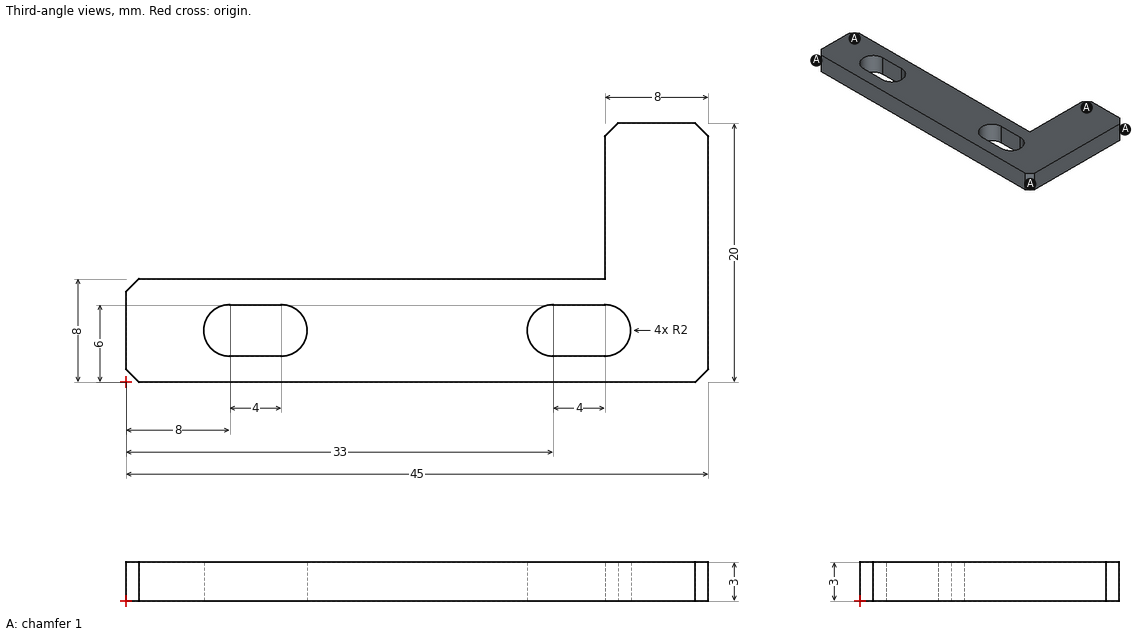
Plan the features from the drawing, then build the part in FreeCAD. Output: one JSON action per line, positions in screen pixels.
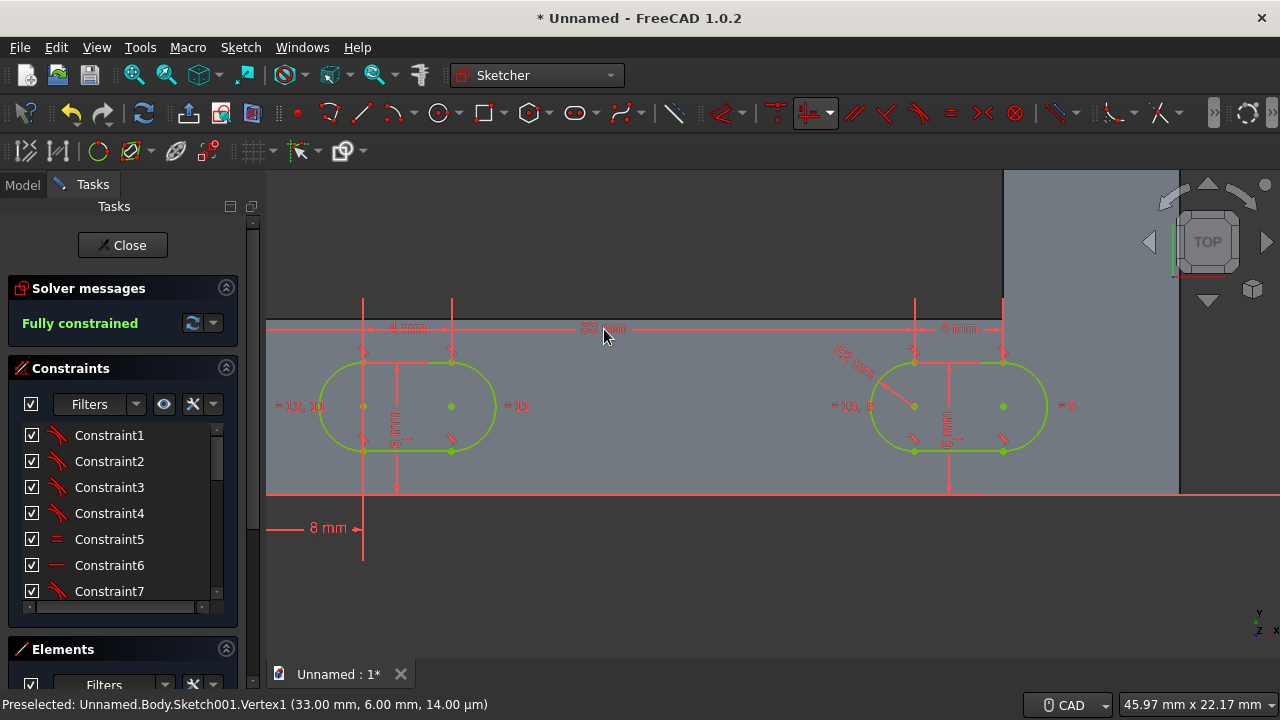
{"action": "left_click", "coordinate": [123, 245]}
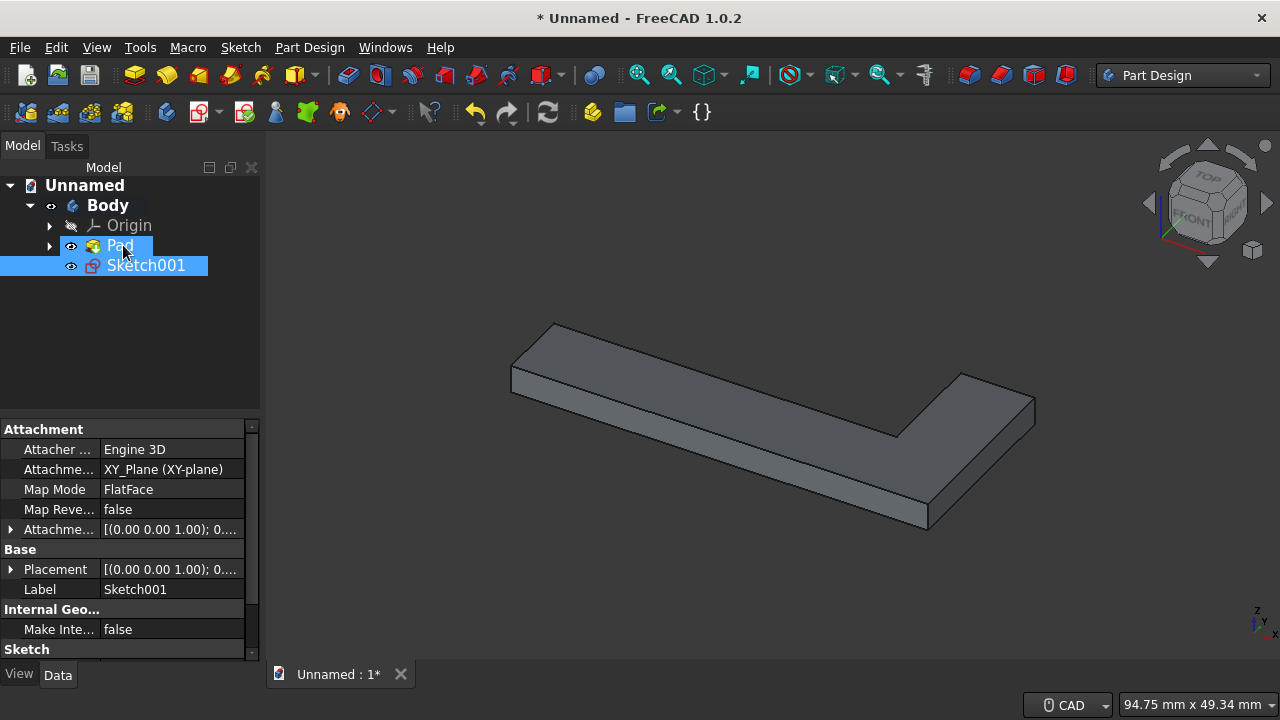
{"action": "left_click", "coordinate": [350, 76]}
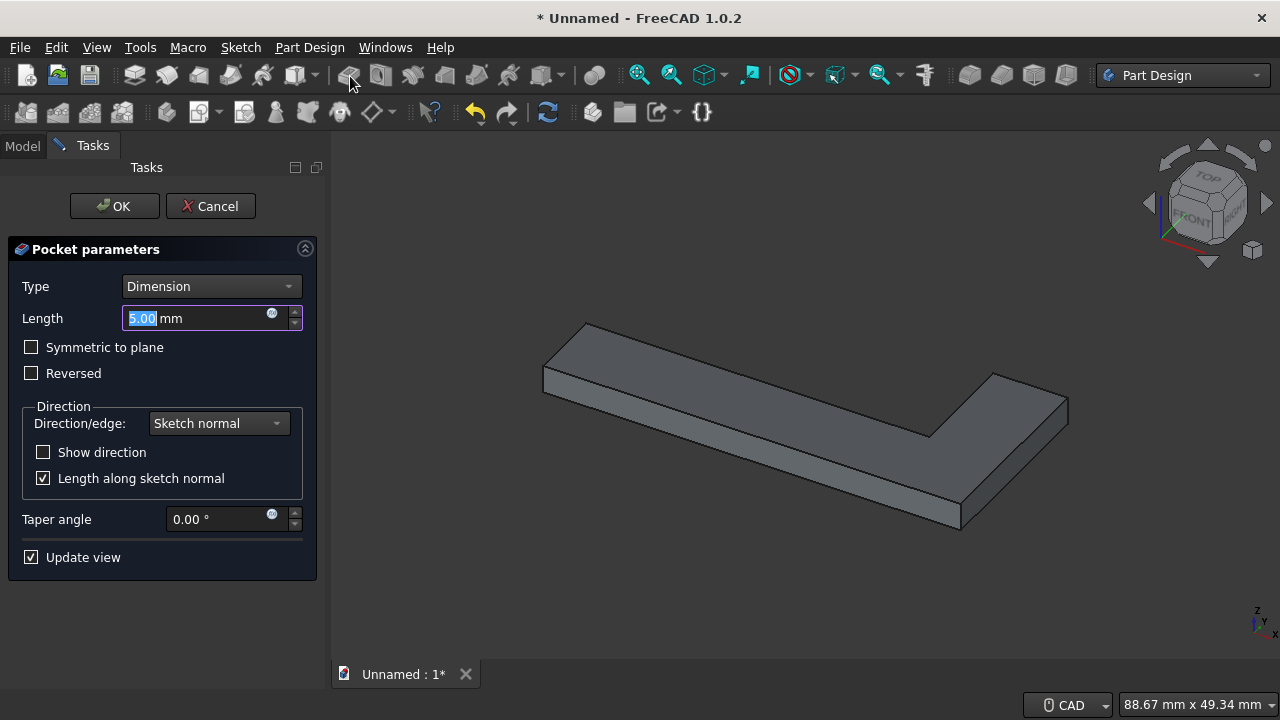
{"action": "type", "text": "3"}
{"action": "key", "text": "Tab"}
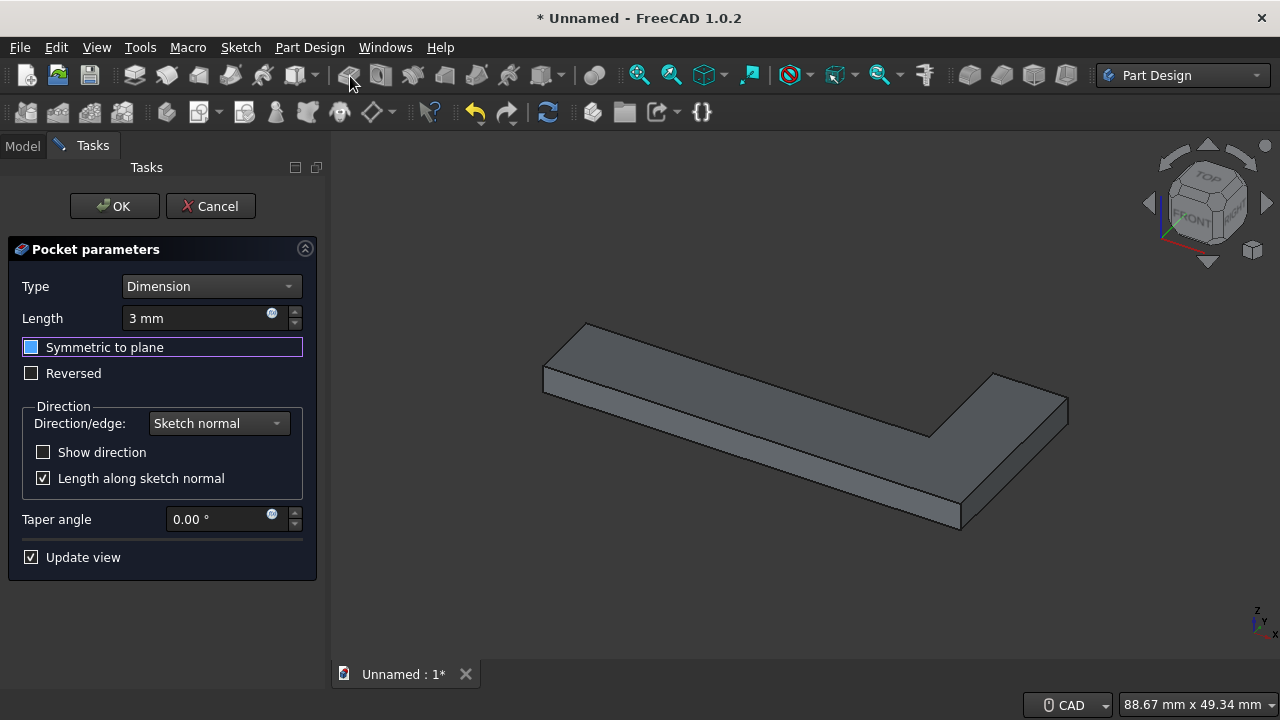
{"action": "left_click", "coordinate": [30, 373]}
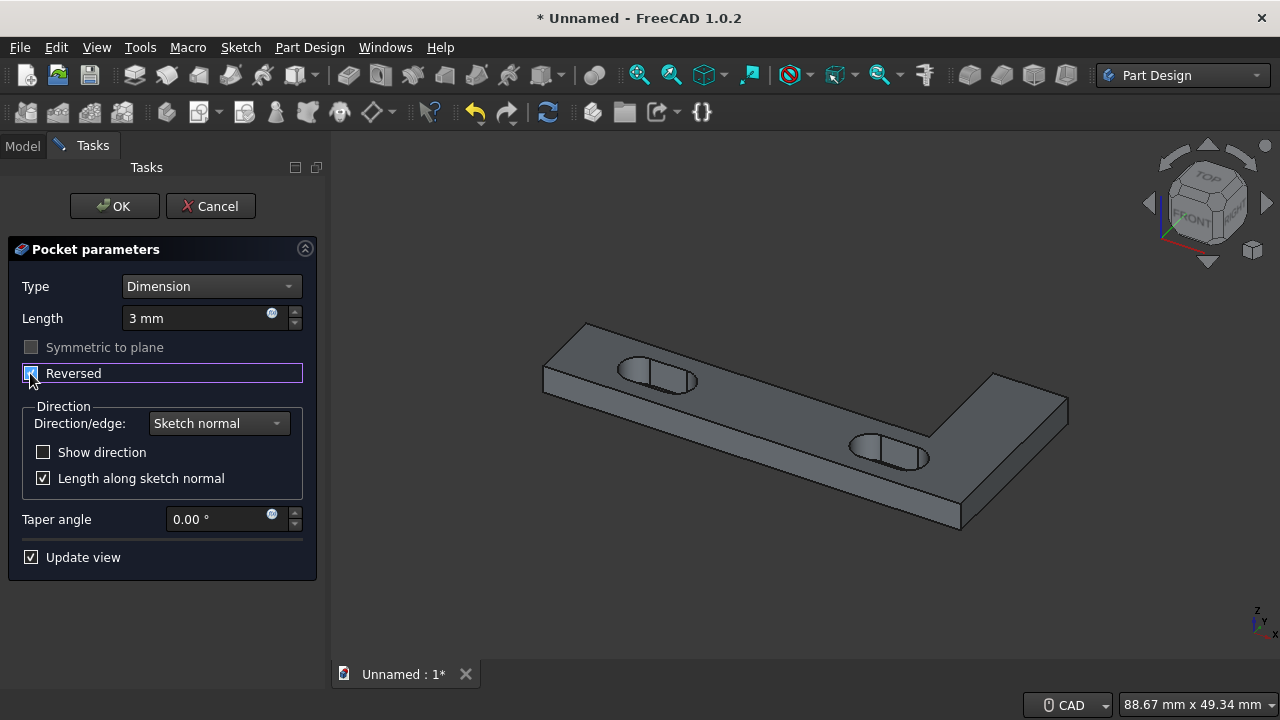
{"action": "left_click", "coordinate": [115, 206]}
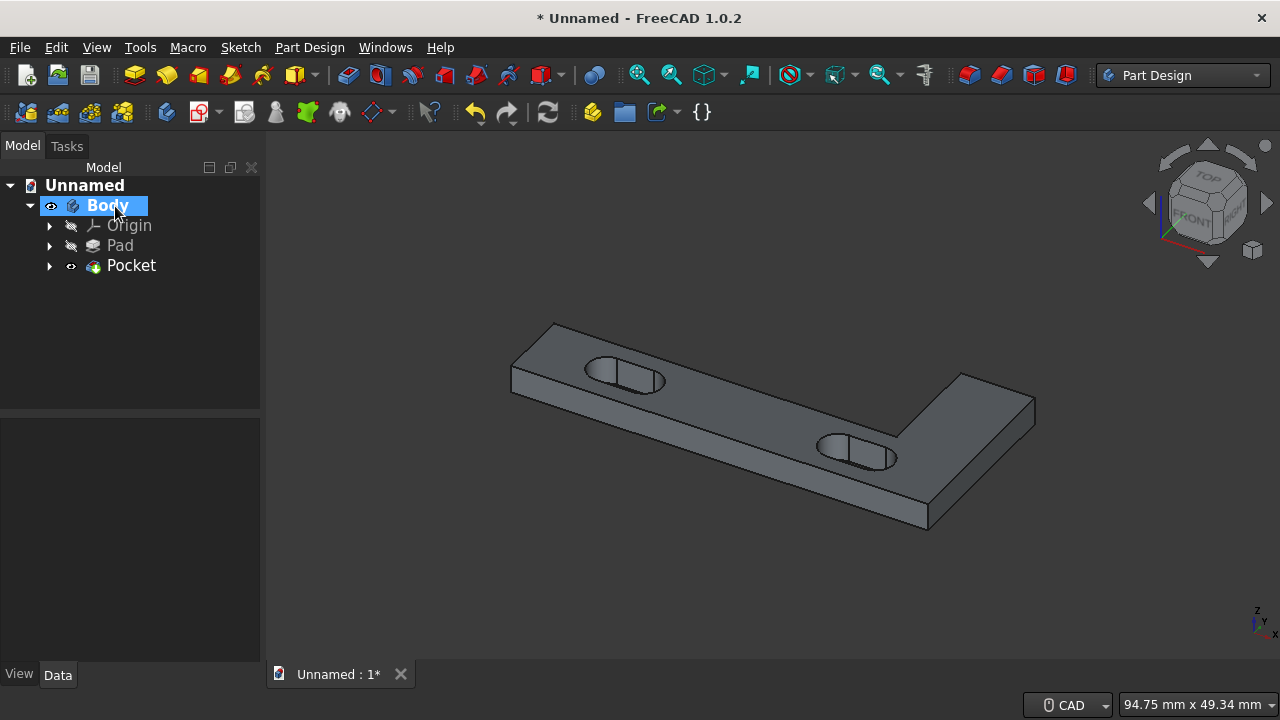
{"action": "left_click", "coordinate": [928, 516]}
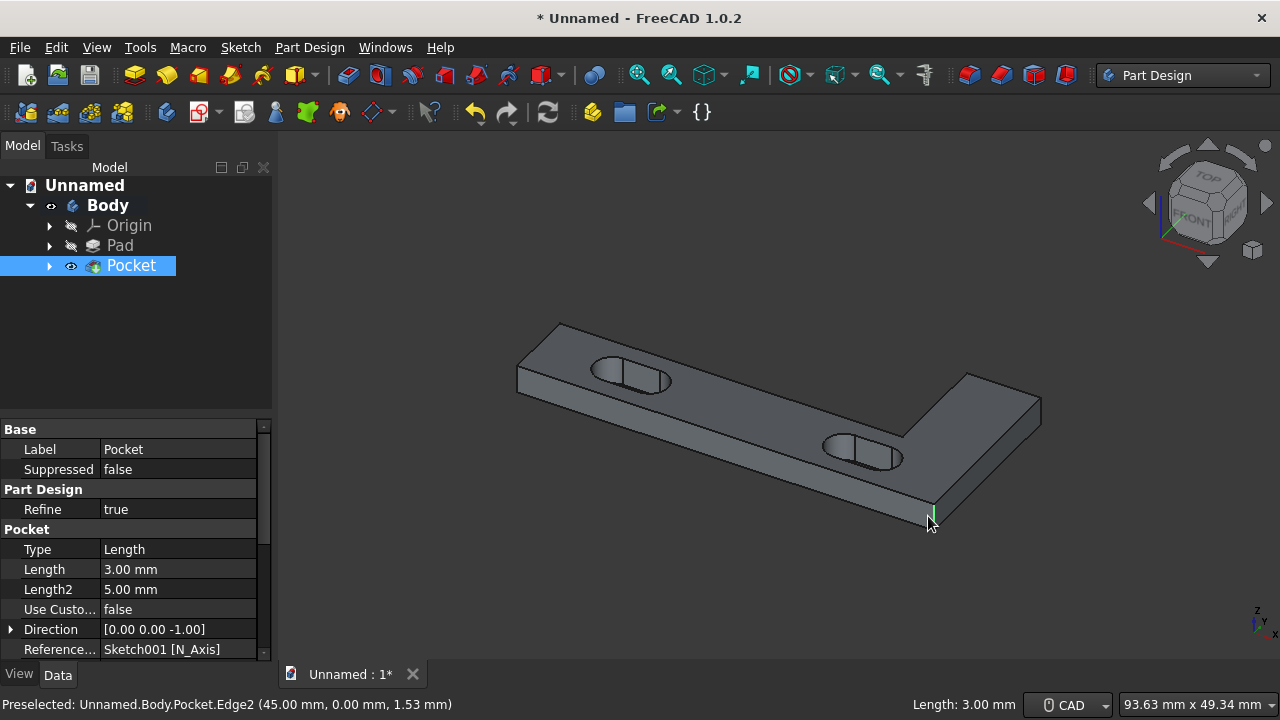
{"action": "key", "text": "0"}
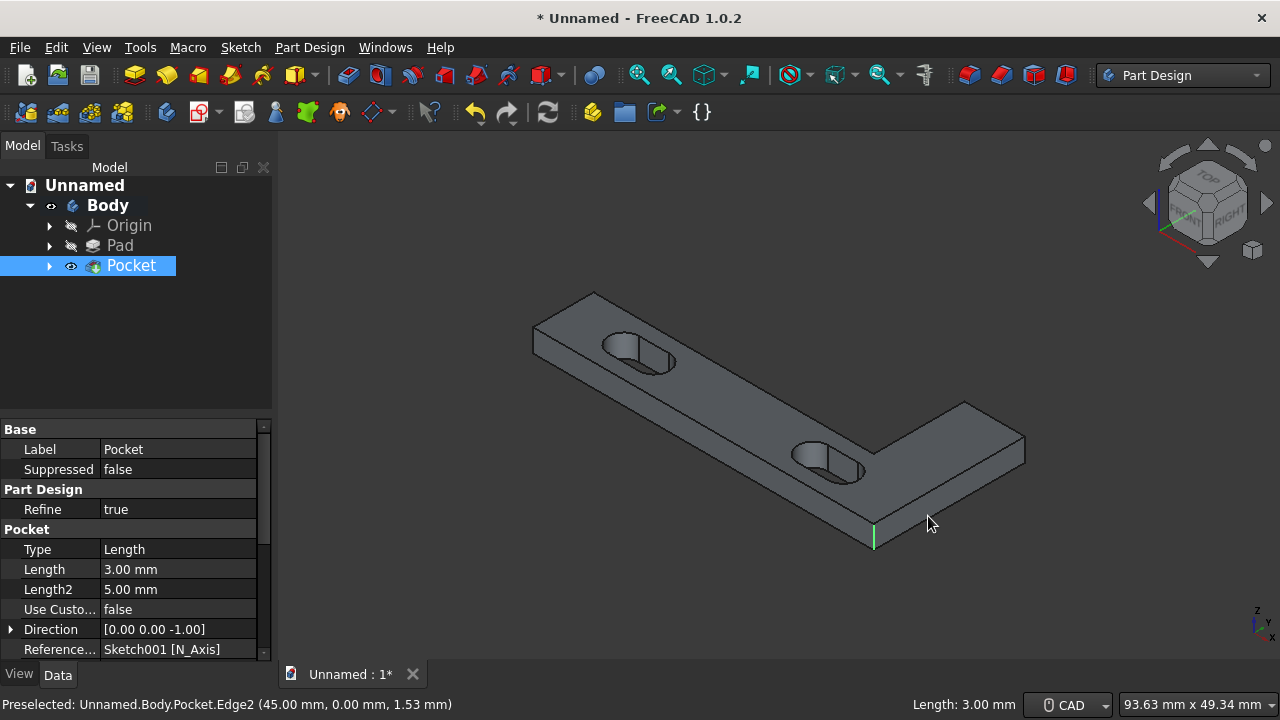
{"action": "key", "text": "2"}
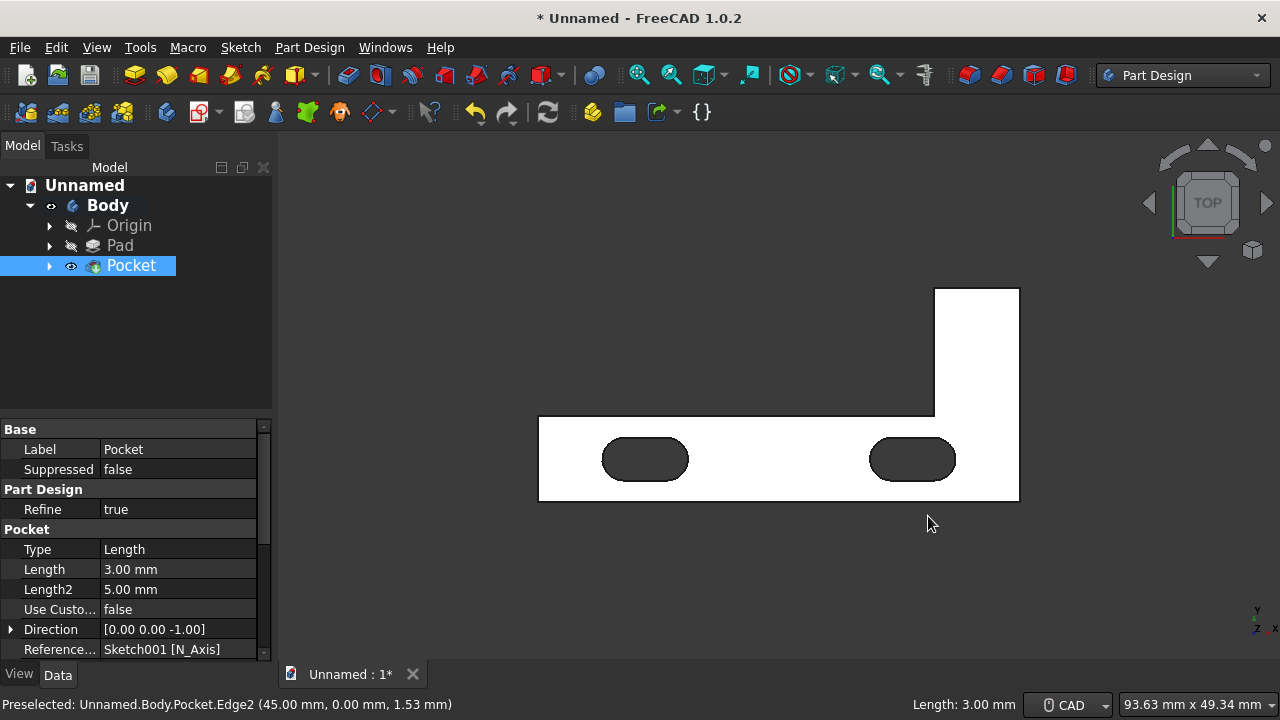
{"action": "key", "text": "1"}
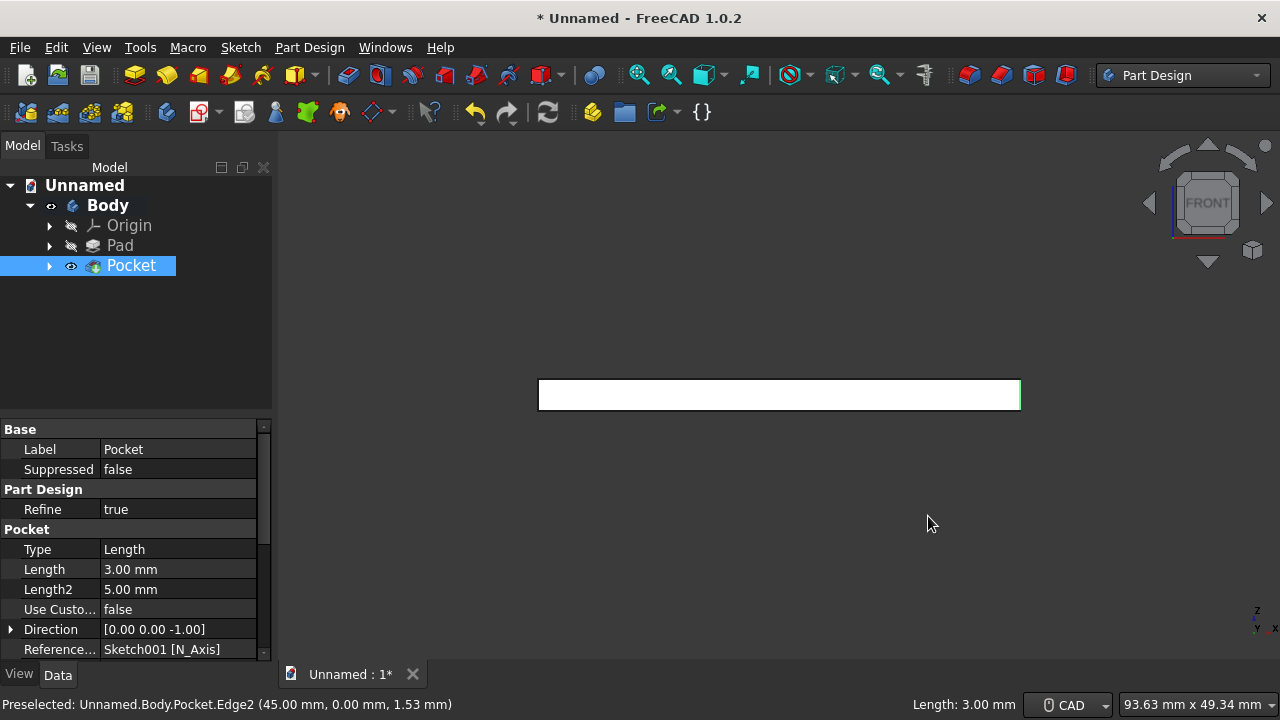
{"action": "left_click", "coordinate": [538, 394], "text": "ctrl"}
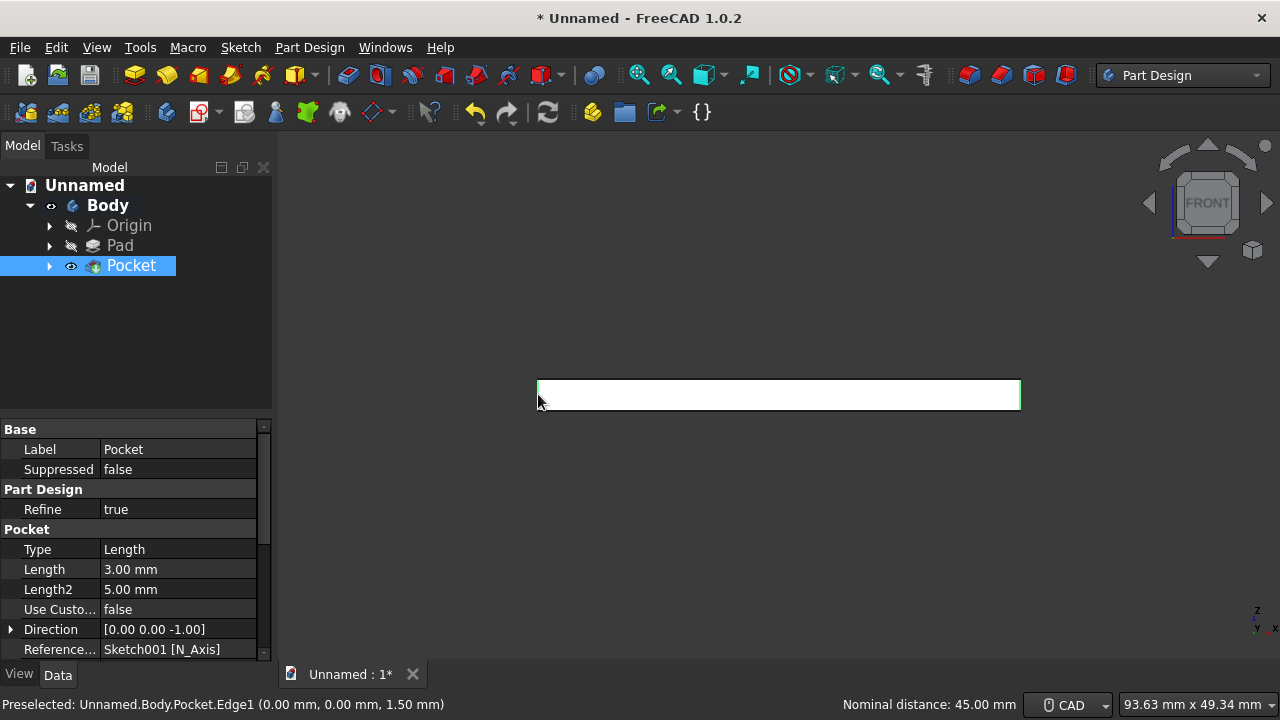
{"action": "key", "text": "3"}